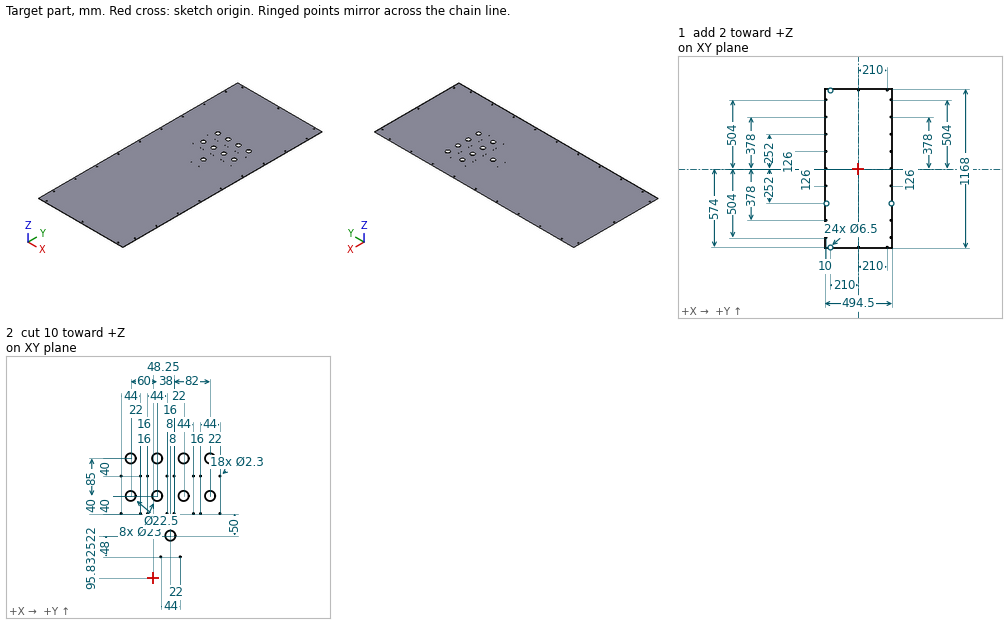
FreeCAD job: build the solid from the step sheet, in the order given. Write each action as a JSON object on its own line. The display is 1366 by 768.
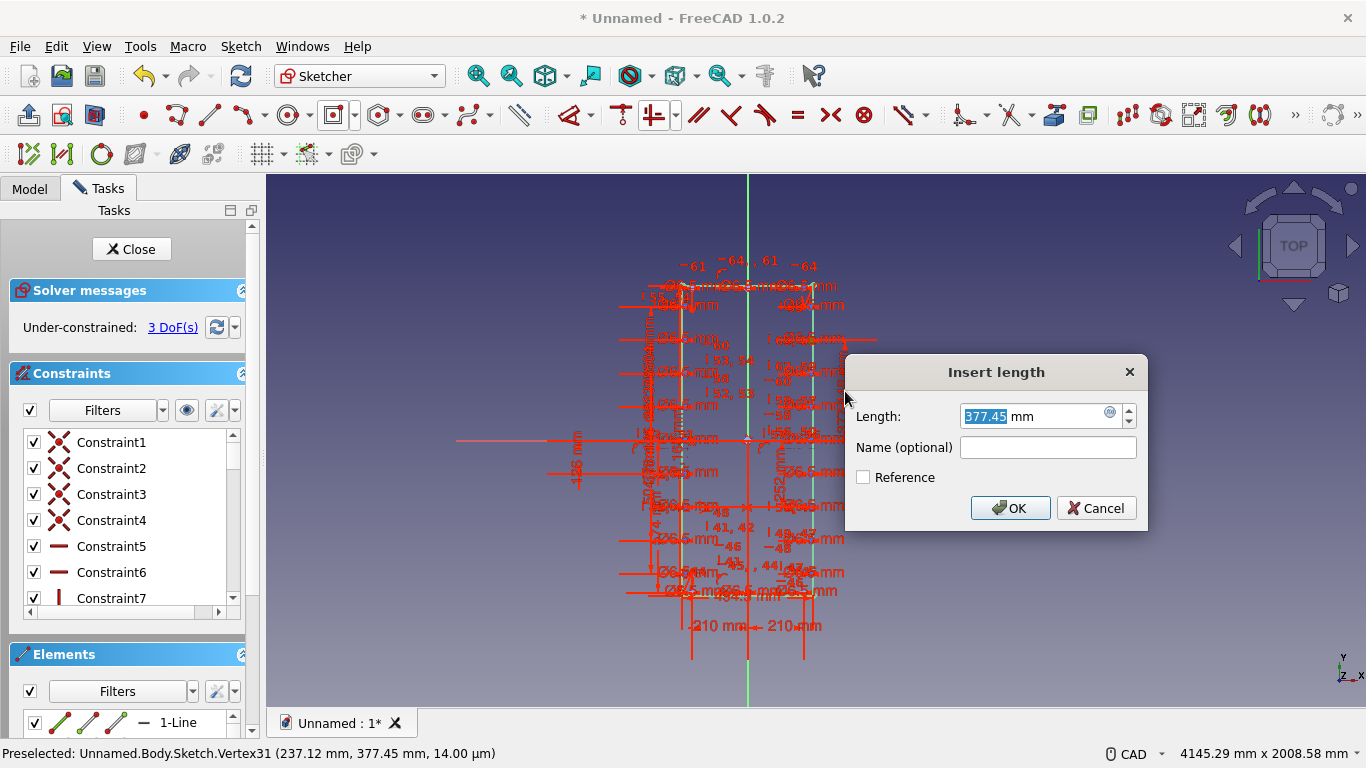
{"action": "type", "text": "378"}
{"action": "key", "text": "Return"}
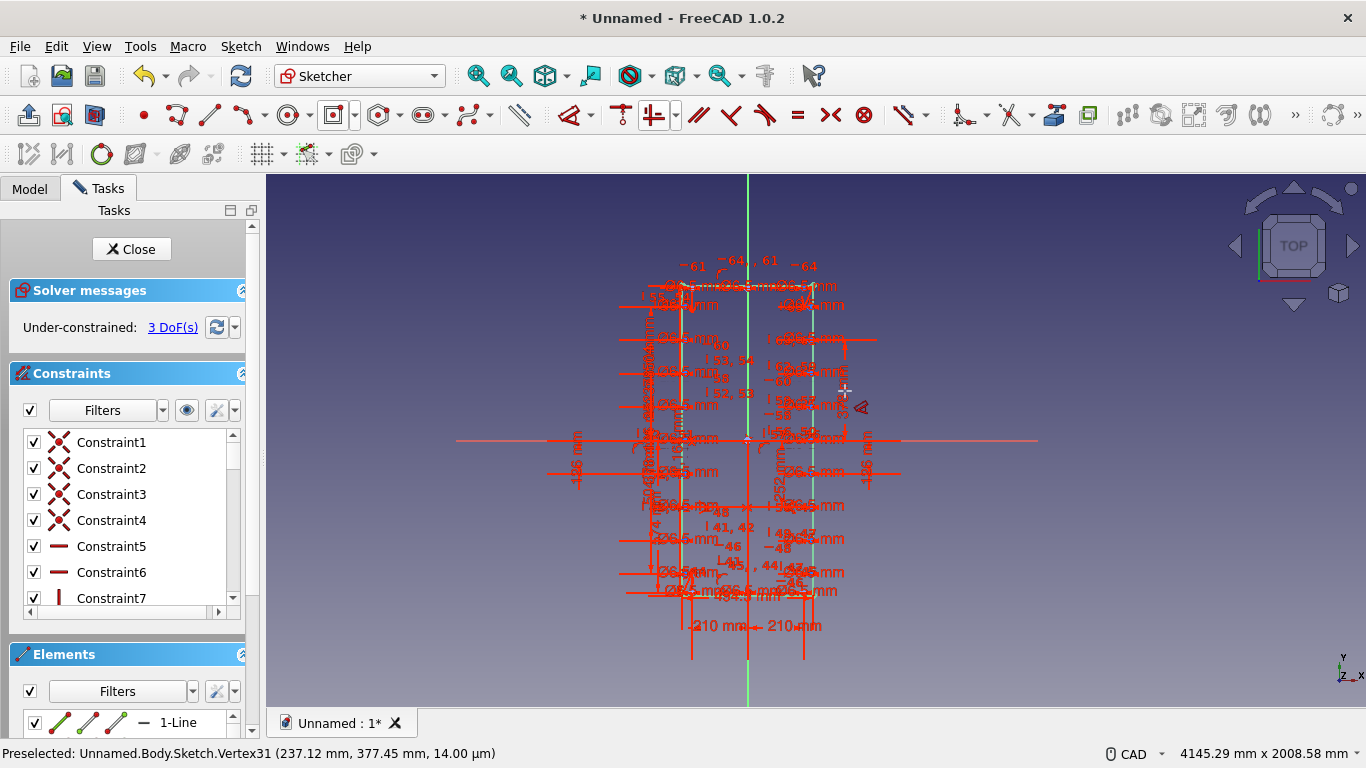
{"action": "left_click", "coordinate": [811, 307]}
{"action": "left_click", "coordinate": [845, 343]}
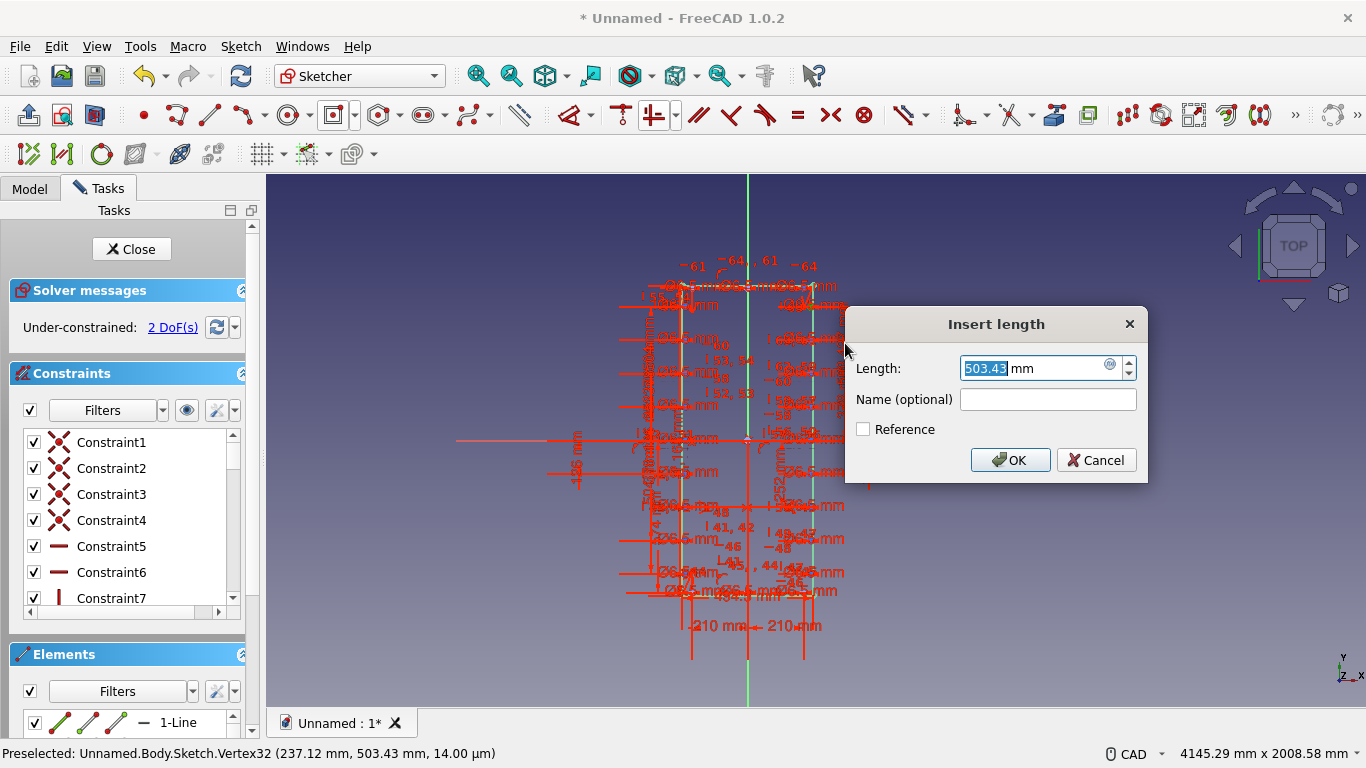
{"action": "type", "text": "504"}
{"action": "key", "text": "Return"}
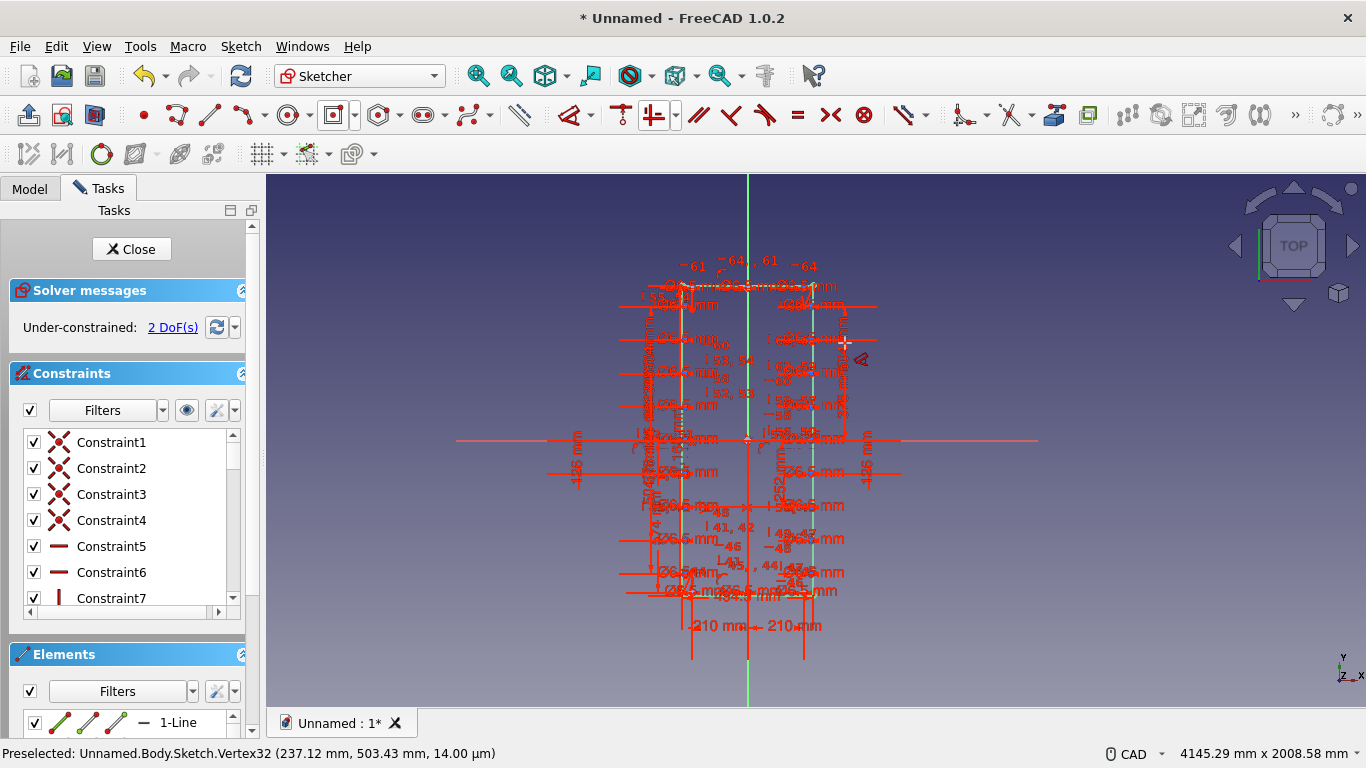
{"action": "left_click", "coordinate": [804, 288]}
{"action": "left_click", "coordinate": [776, 254]}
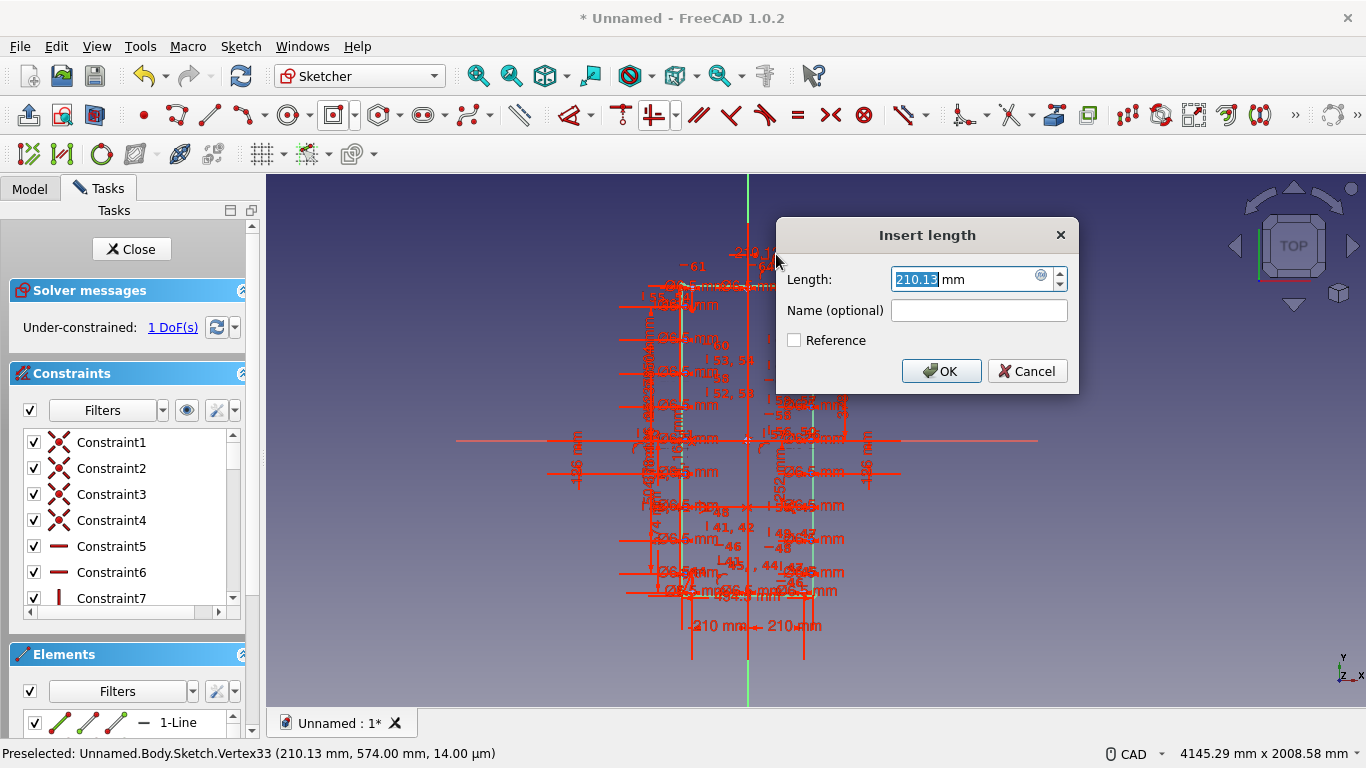
{"action": "type", "text": "210"}
{"action": "key", "text": "Return"}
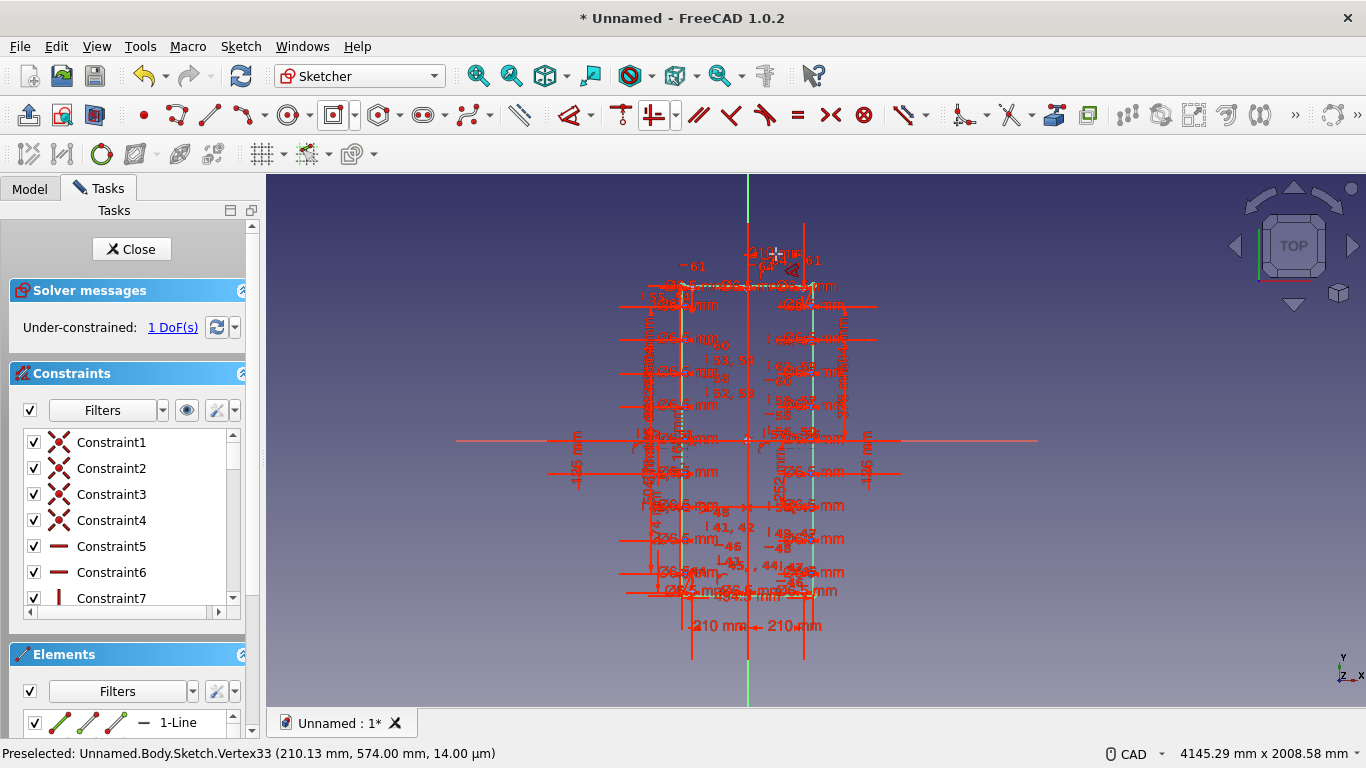
{"action": "scroll", "coordinate": [682, 596], "scroll_direction": "up", "scroll_amount": 14}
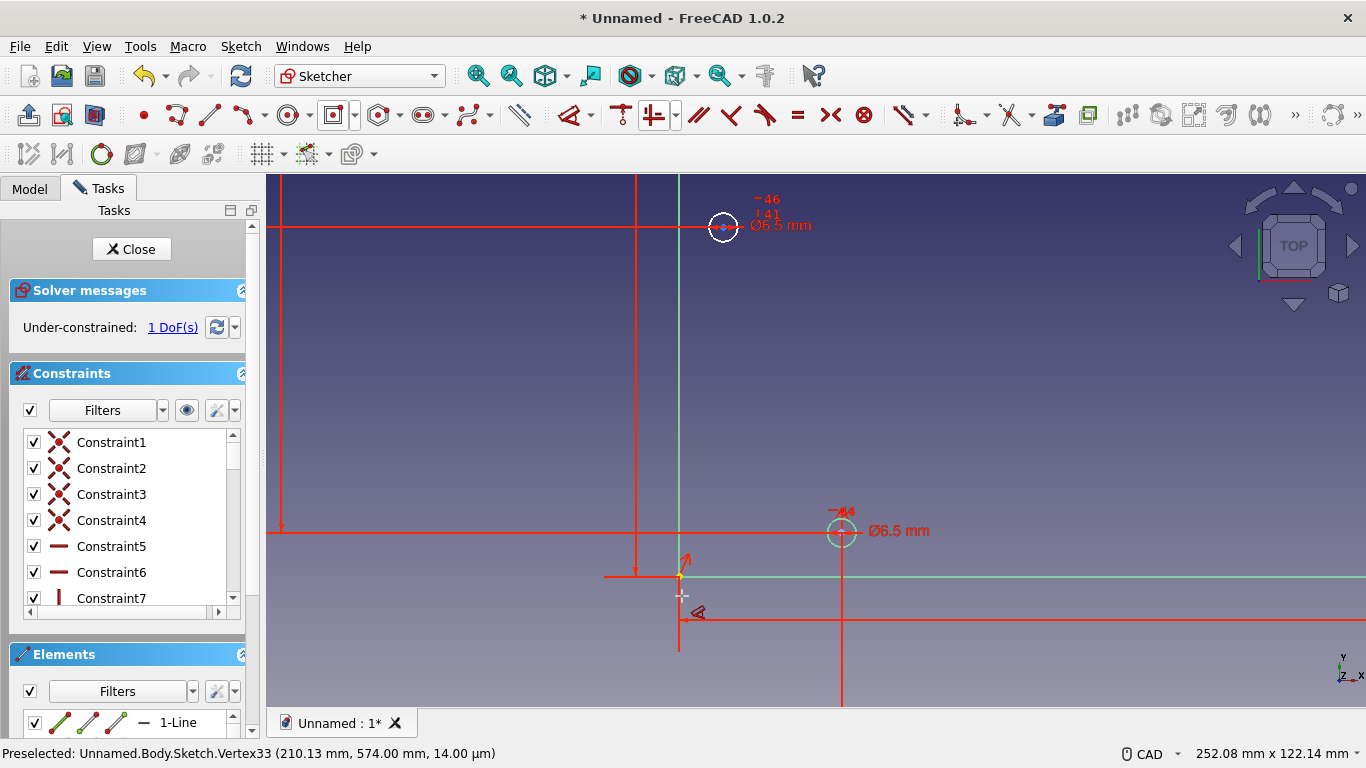
{"action": "left_click", "coordinate": [679, 577]}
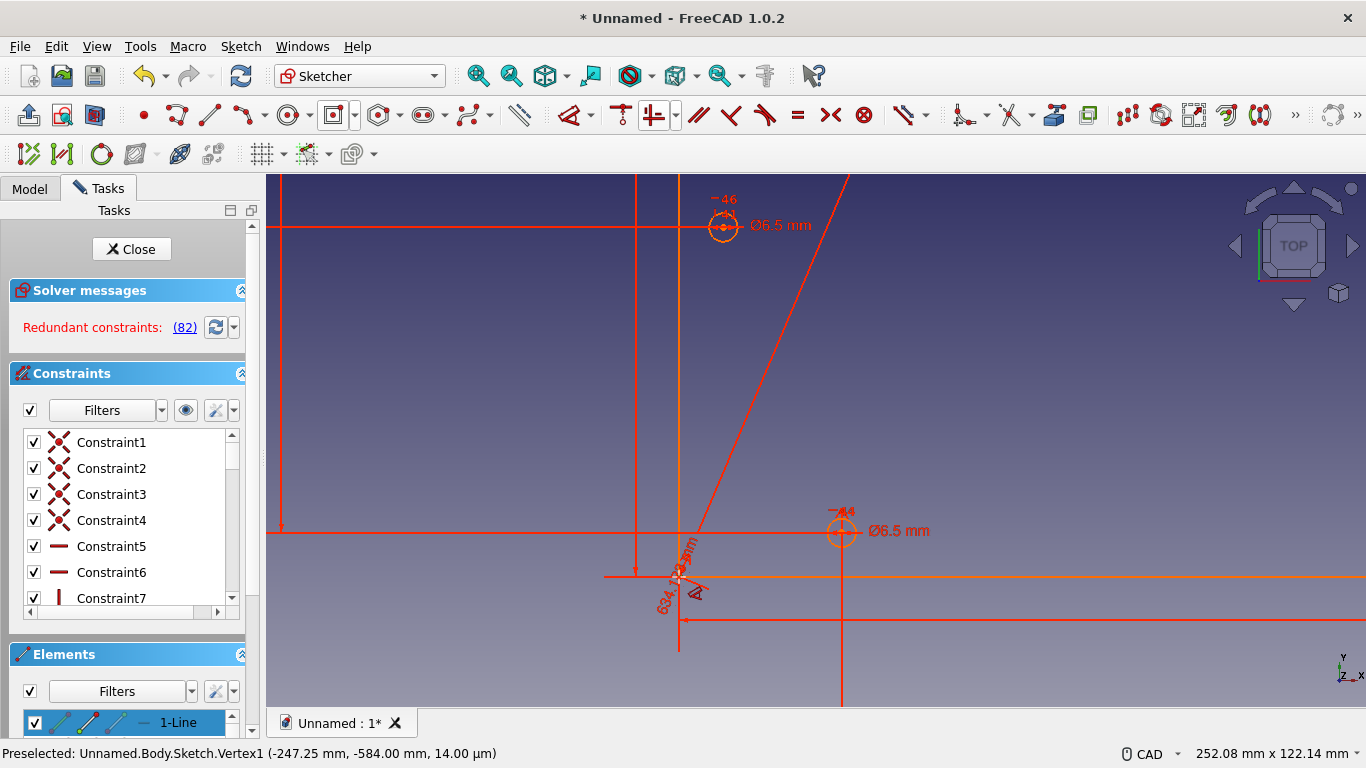
{"action": "left_click", "coordinate": [723, 227]}
{"action": "left_click", "coordinate": [701, 611]}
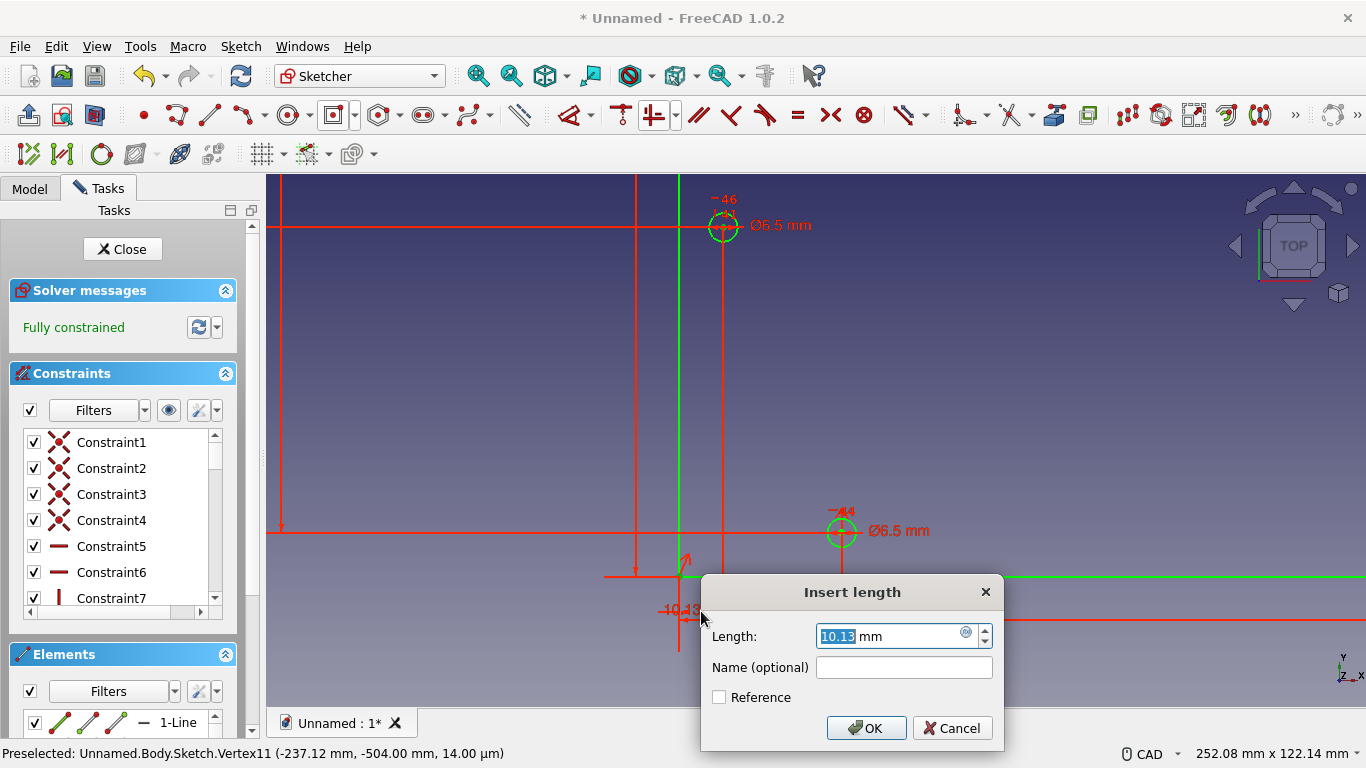
{"action": "type", "text": "10"}
{"action": "key", "text": "Return"}
{"action": "key", "text": "Escape"}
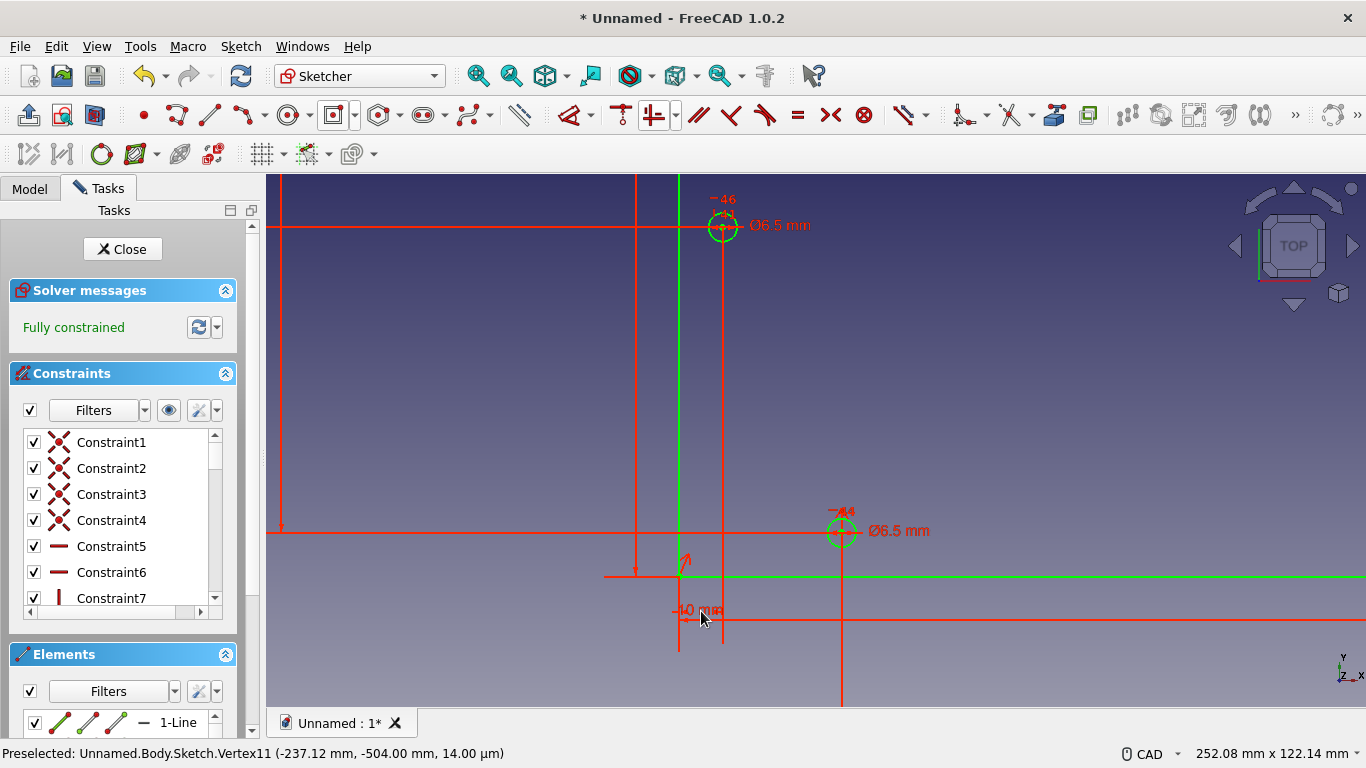
{"action": "left_click", "coordinate": [123, 249]}